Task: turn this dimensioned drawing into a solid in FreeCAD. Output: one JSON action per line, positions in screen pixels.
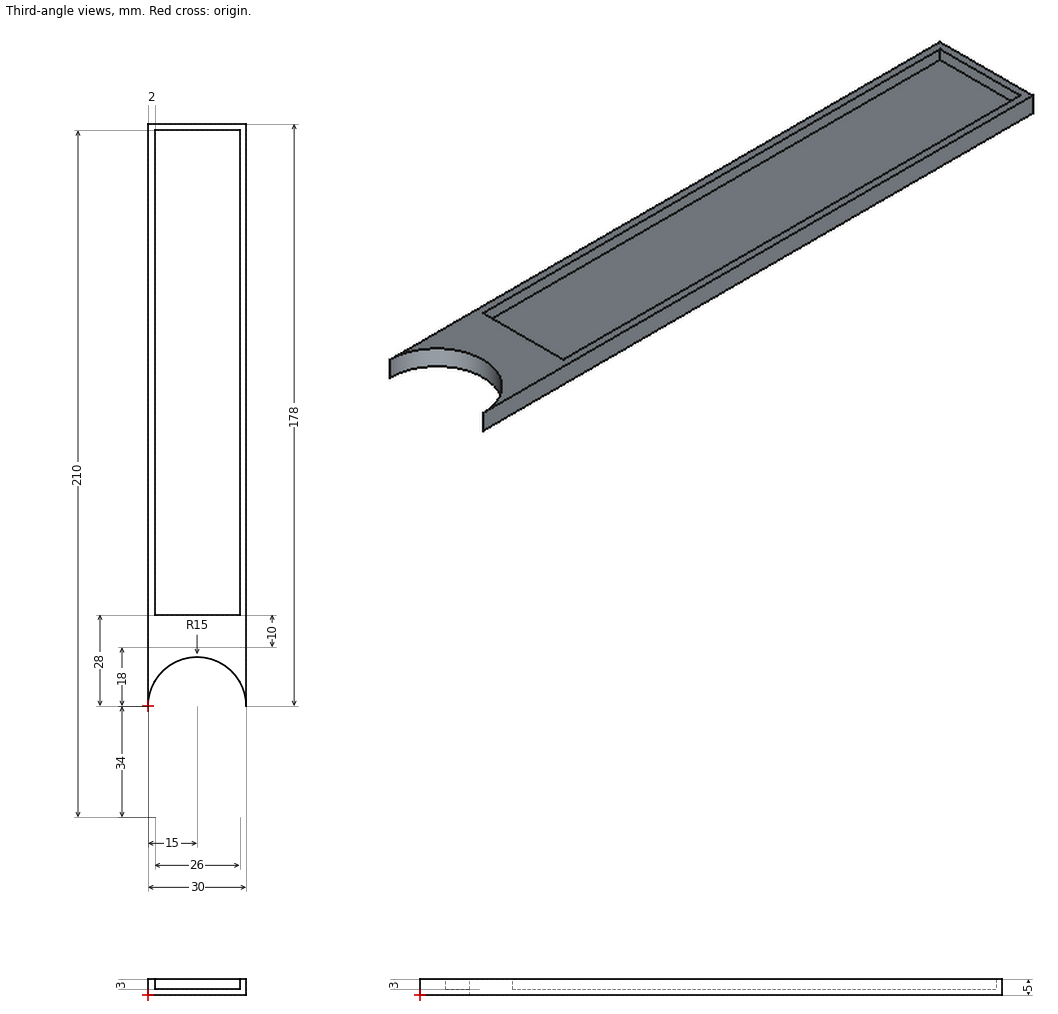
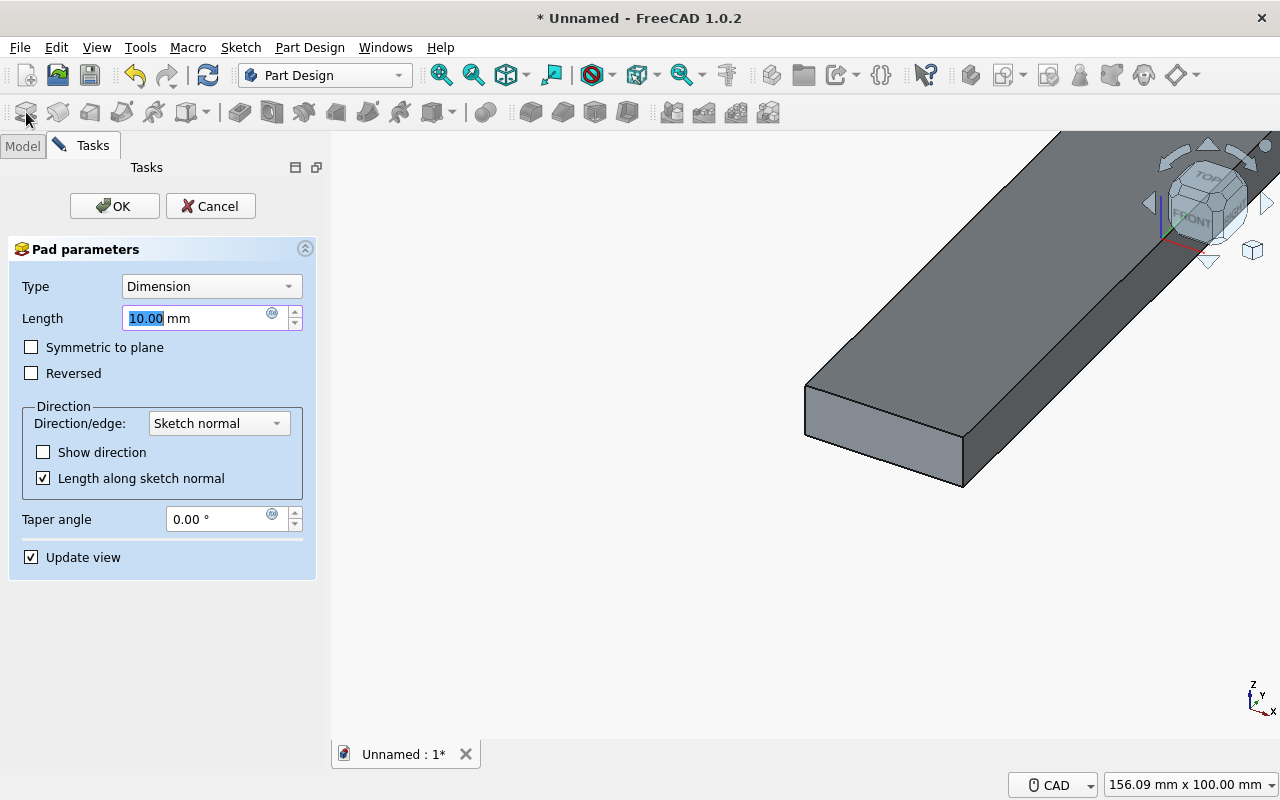
{"action": "type", "text": "5"}
{"action": "key", "text": "Tab"}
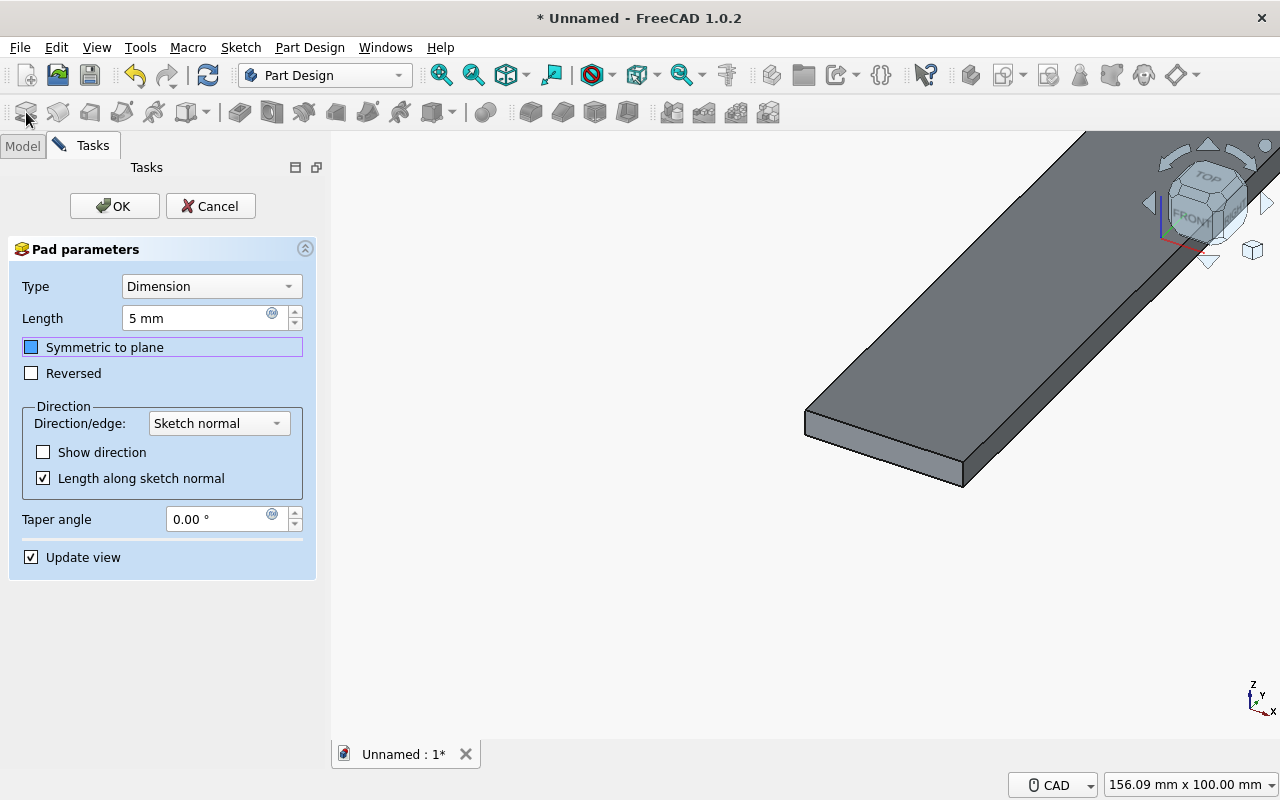
{"action": "left_click", "coordinate": [115, 206]}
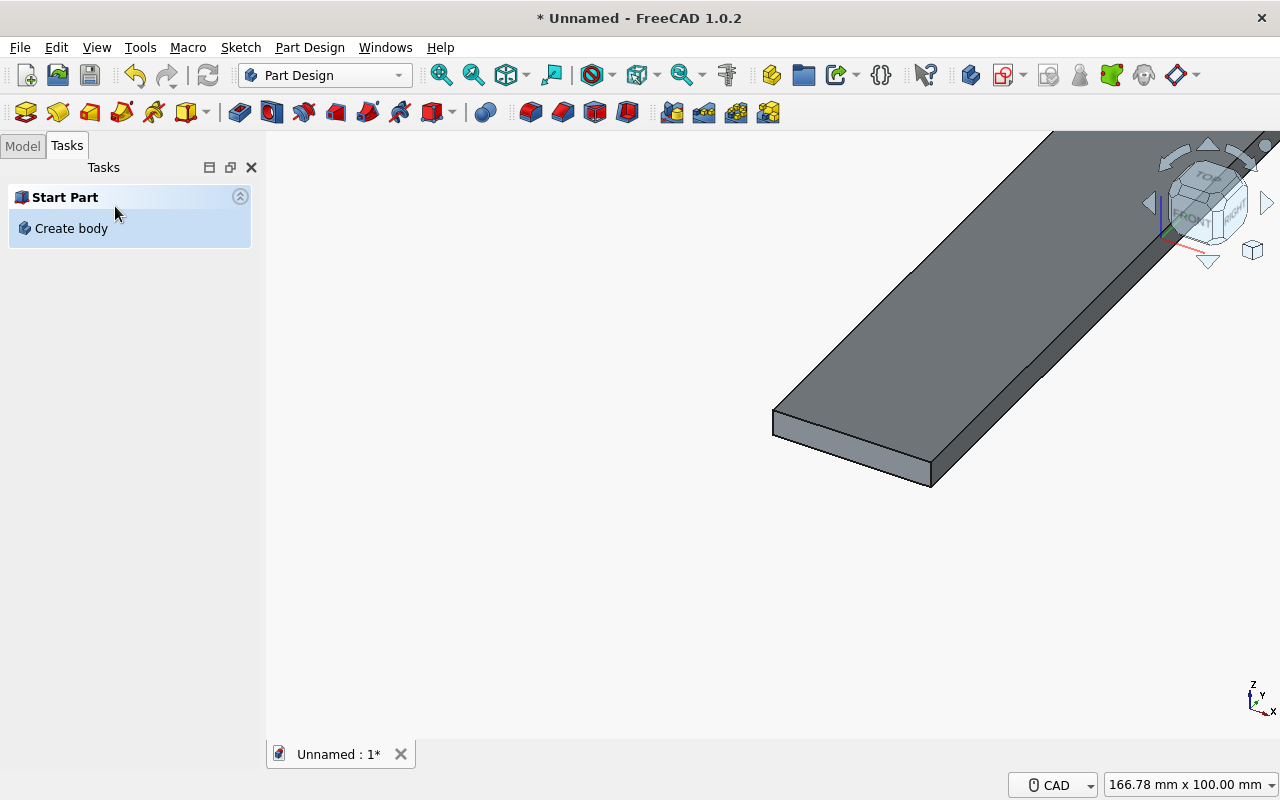
{"action": "left_click", "coordinate": [442, 76]}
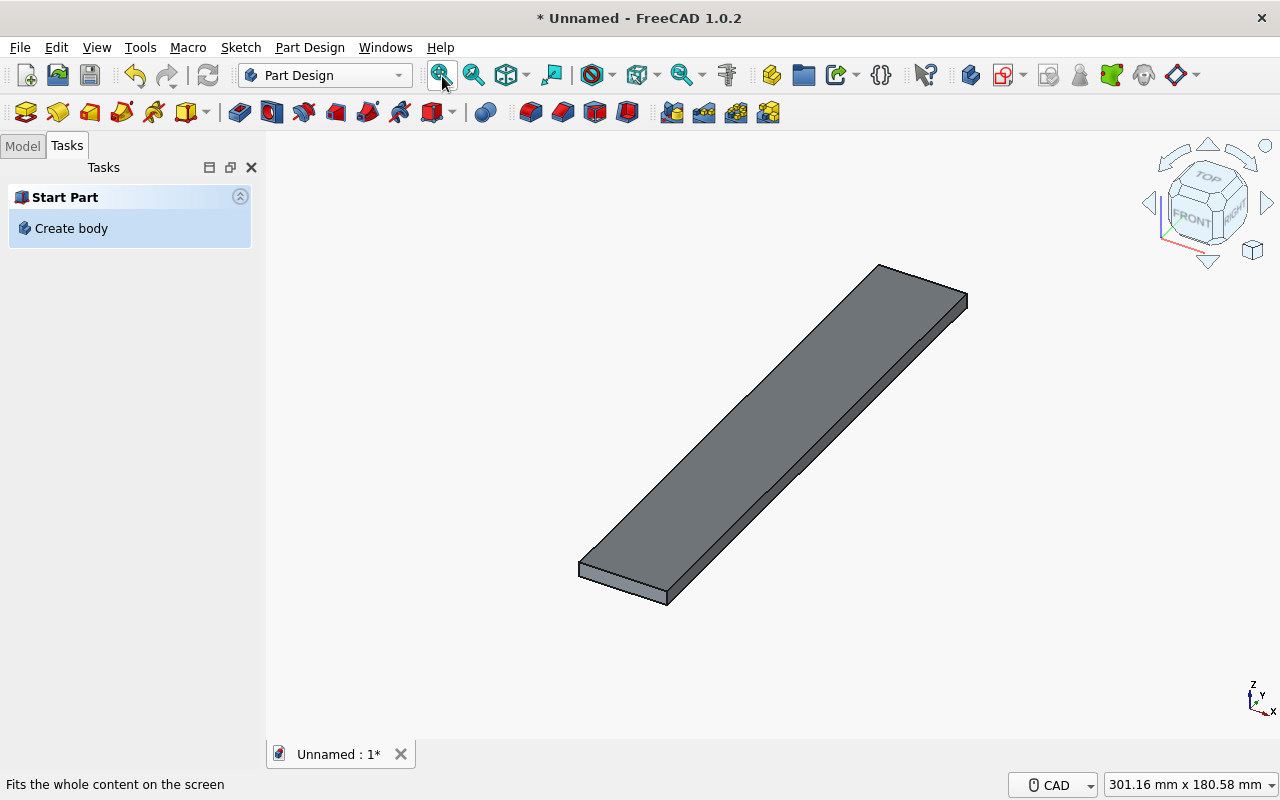
{"action": "left_click", "coordinate": [859, 342]}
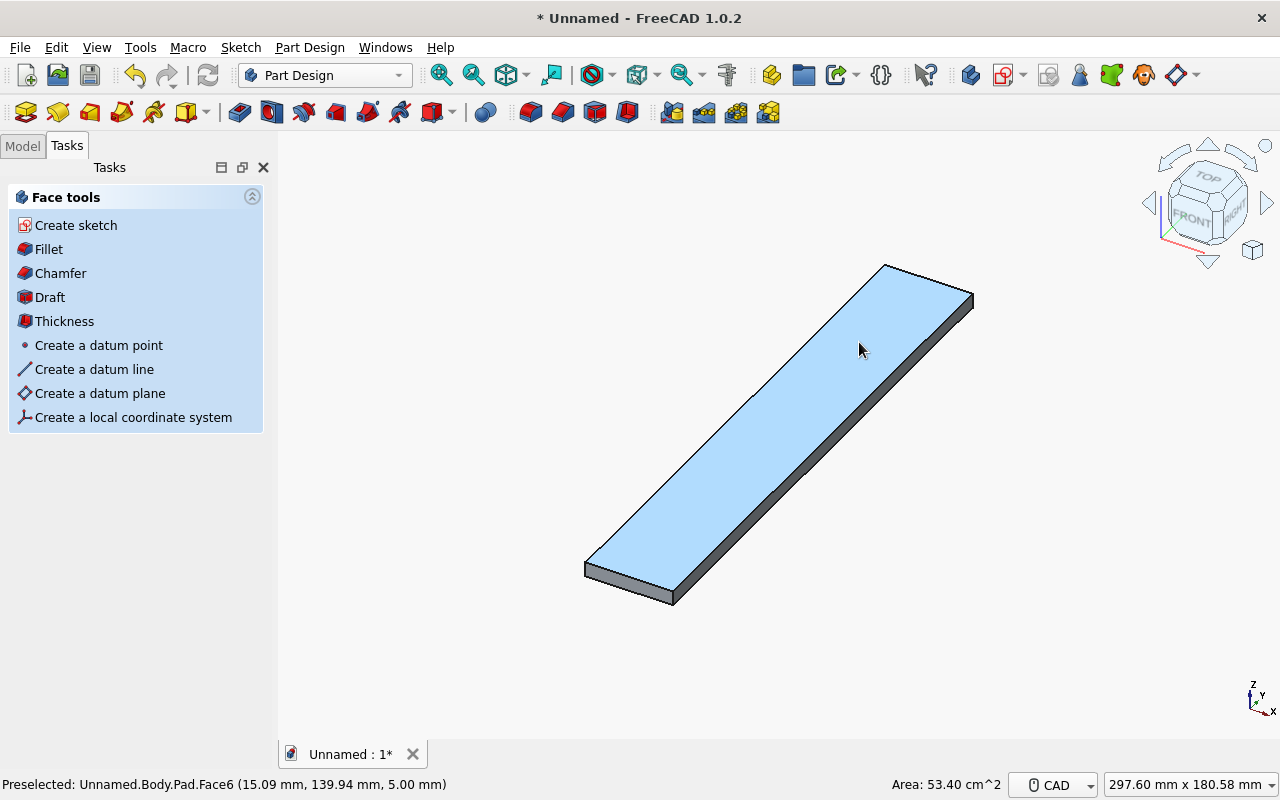
{"action": "left_click", "coordinate": [1004, 76]}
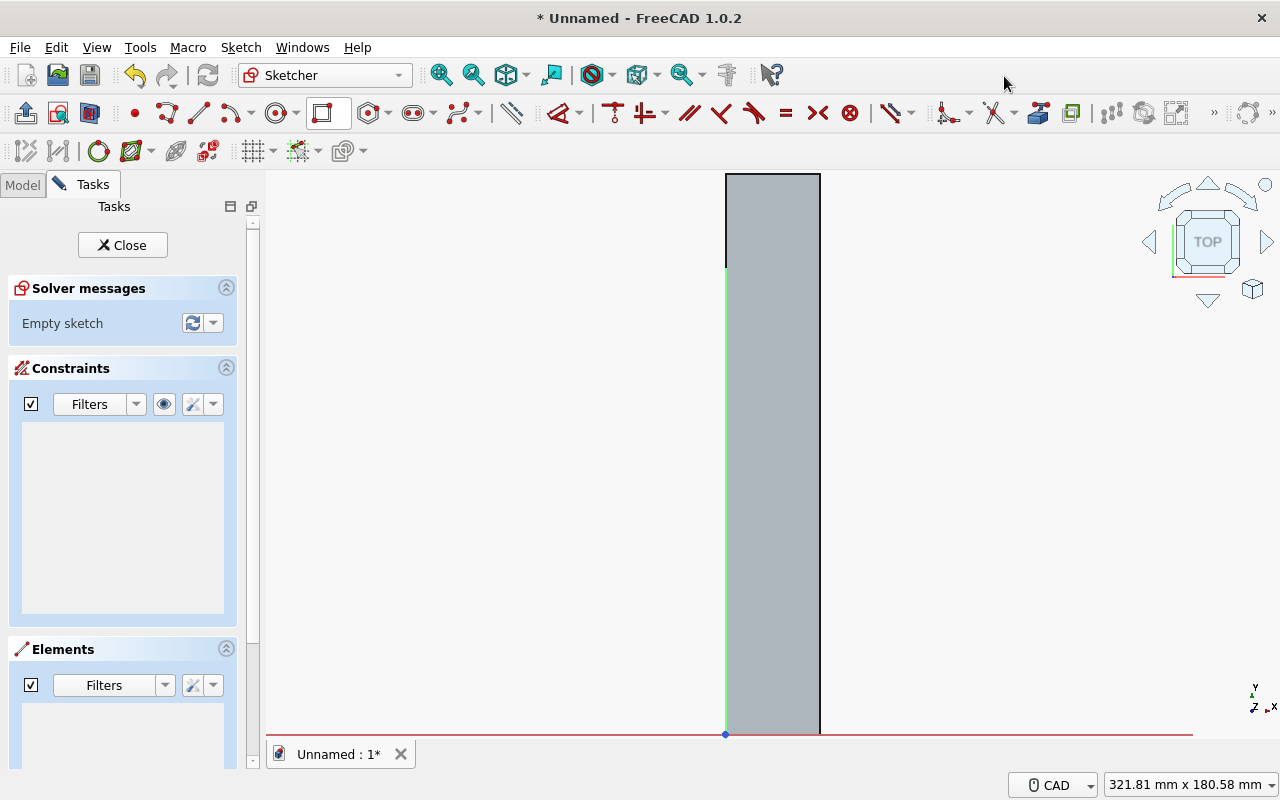
{"action": "scroll", "coordinate": [625, 386], "scroll_direction": "down", "scroll_amount": 3}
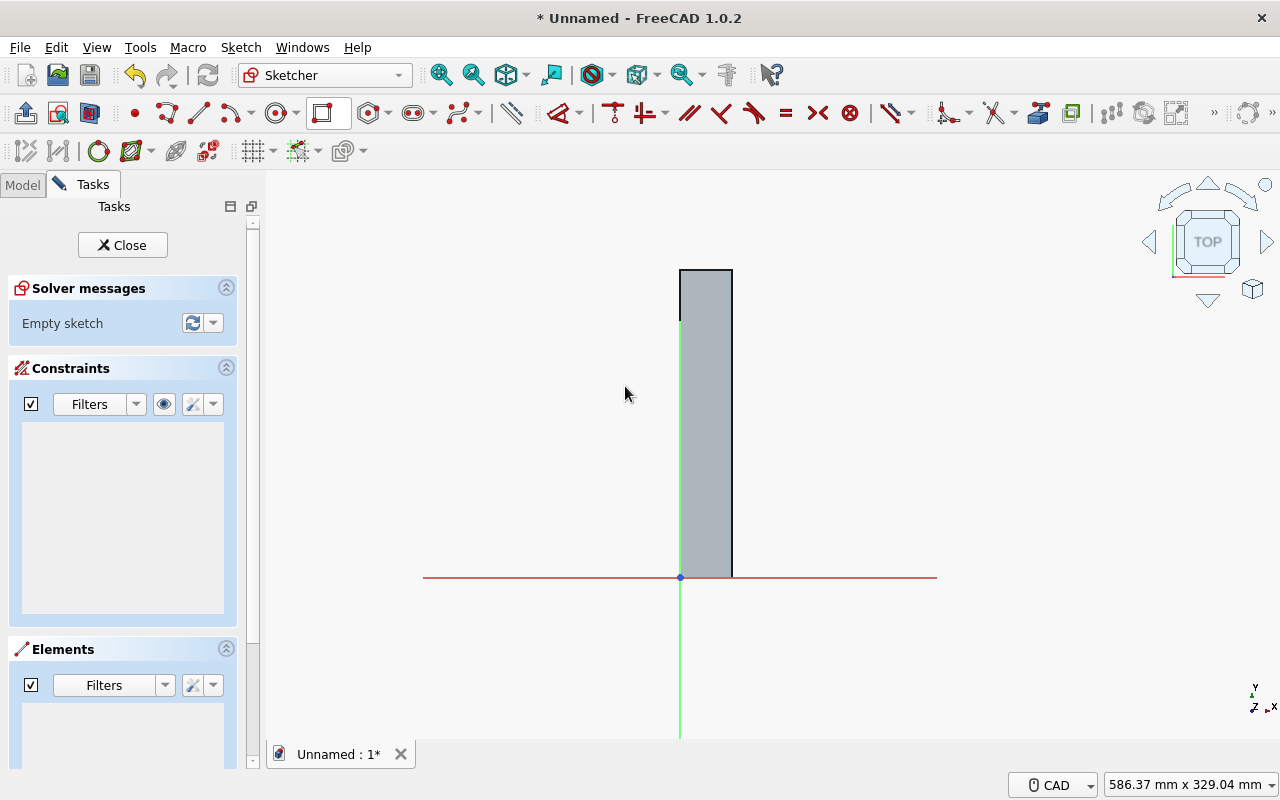
{"action": "key", "text": "g r"}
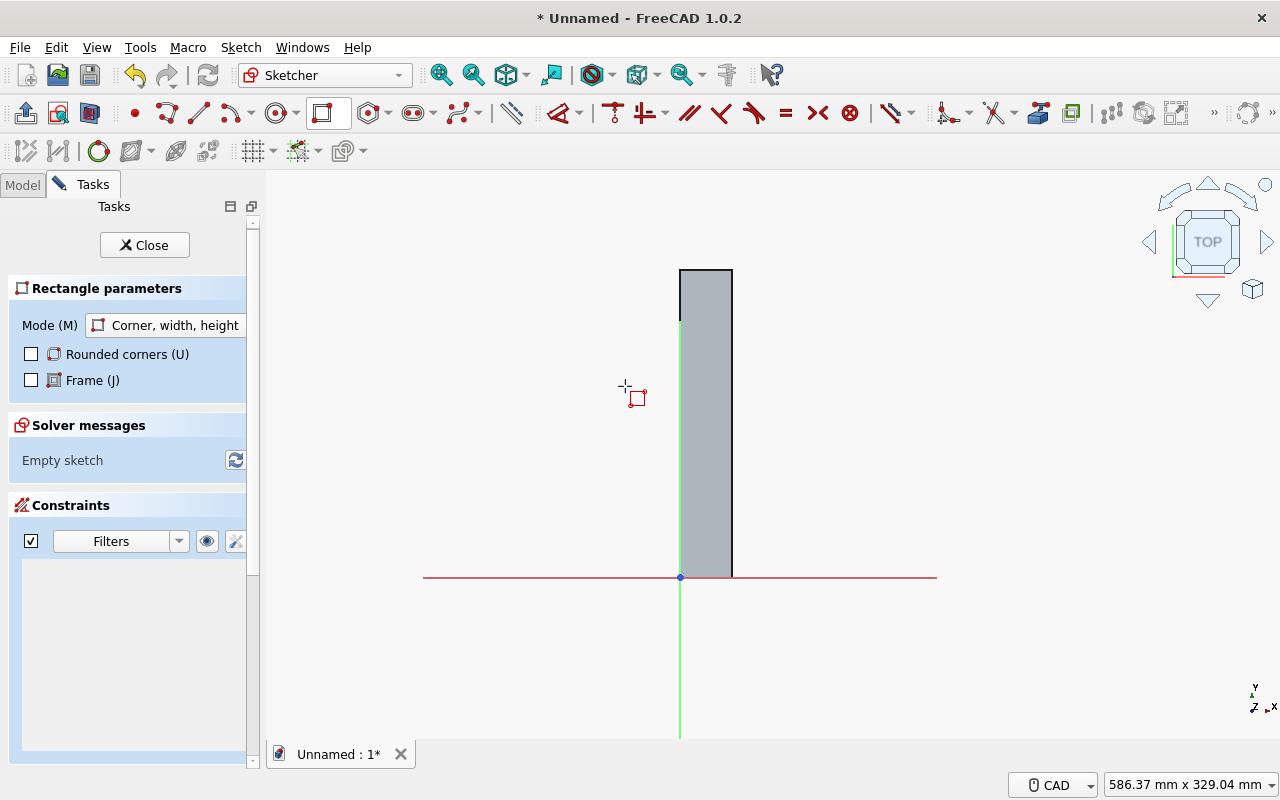
{"action": "scroll", "coordinate": [684, 273], "scroll_direction": "up", "scroll_amount": 8}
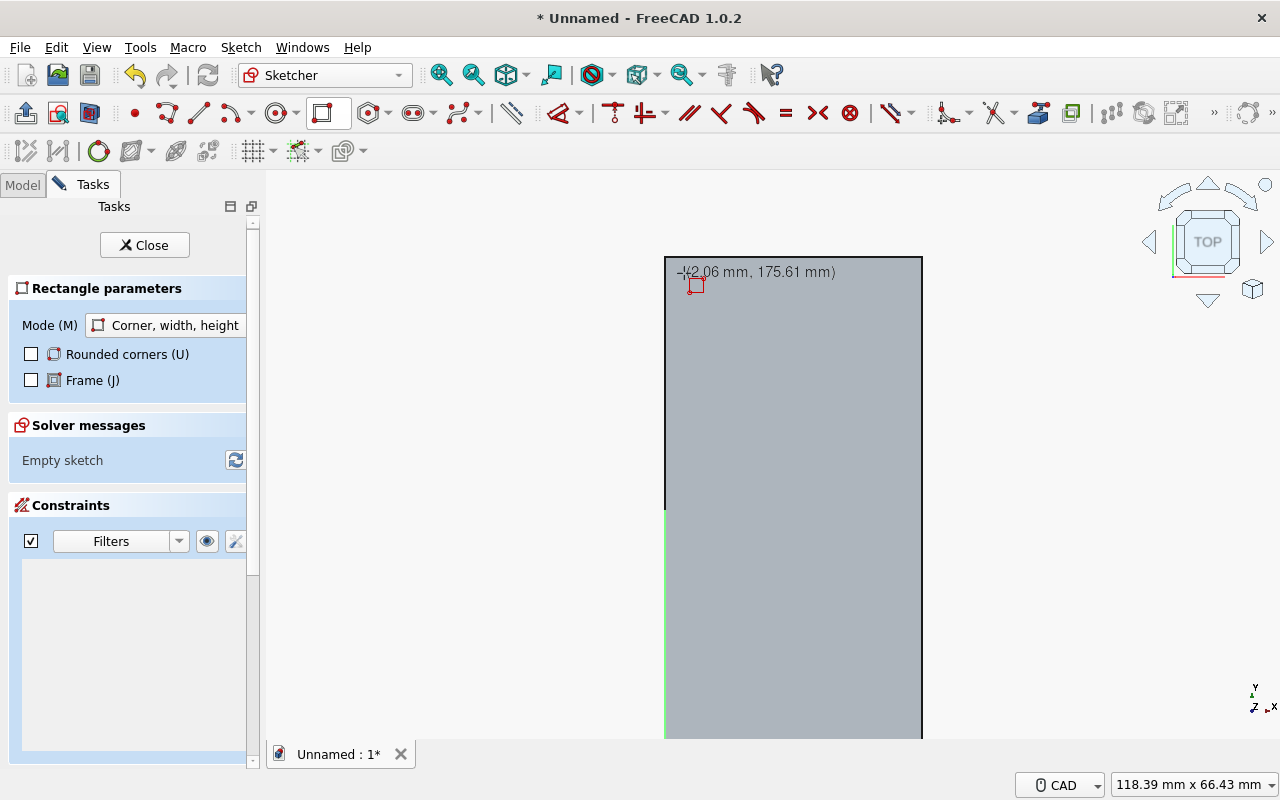
{"action": "left_click", "coordinate": [682, 274]}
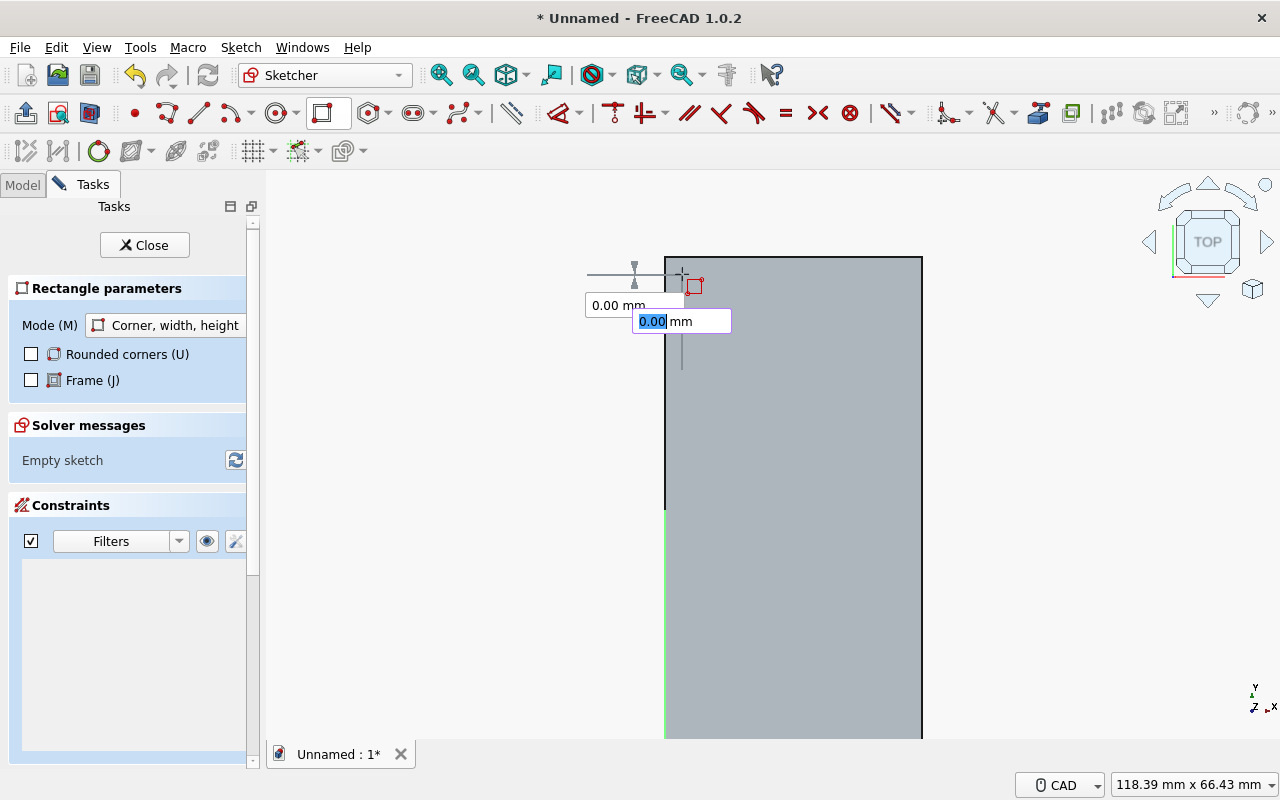
{"action": "scroll", "coordinate": [684, 273], "scroll_direction": "down", "scroll_amount": 8}